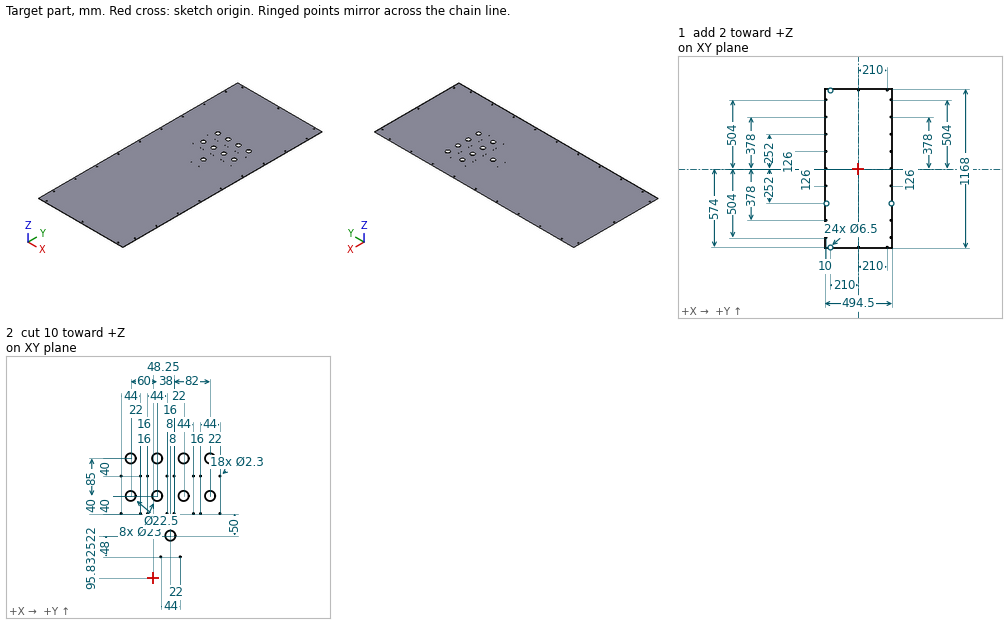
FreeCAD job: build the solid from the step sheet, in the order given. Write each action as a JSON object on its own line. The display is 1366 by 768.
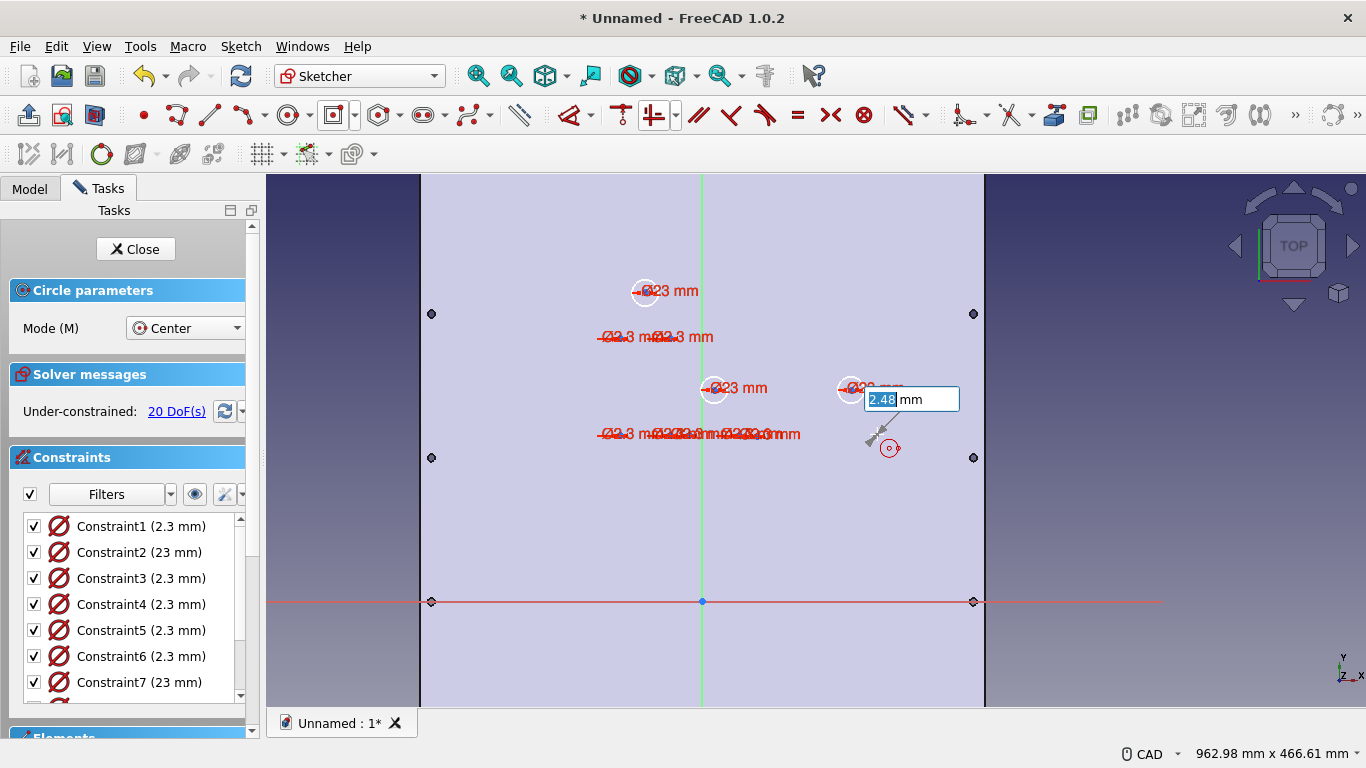
{"action": "type", "text": "2.3"}
{"action": "key", "text": "Return"}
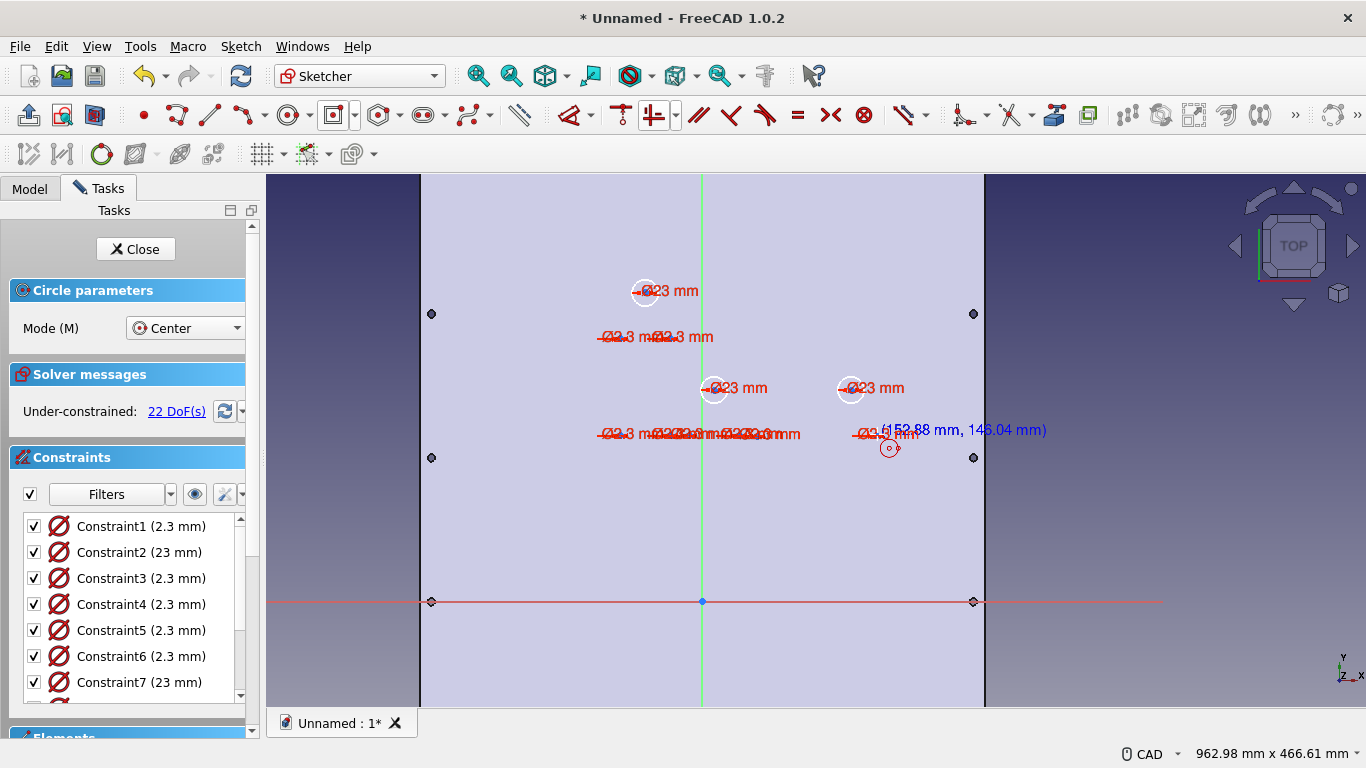
{"action": "scroll", "coordinate": [826, 435], "scroll_direction": "up", "scroll_amount": 15}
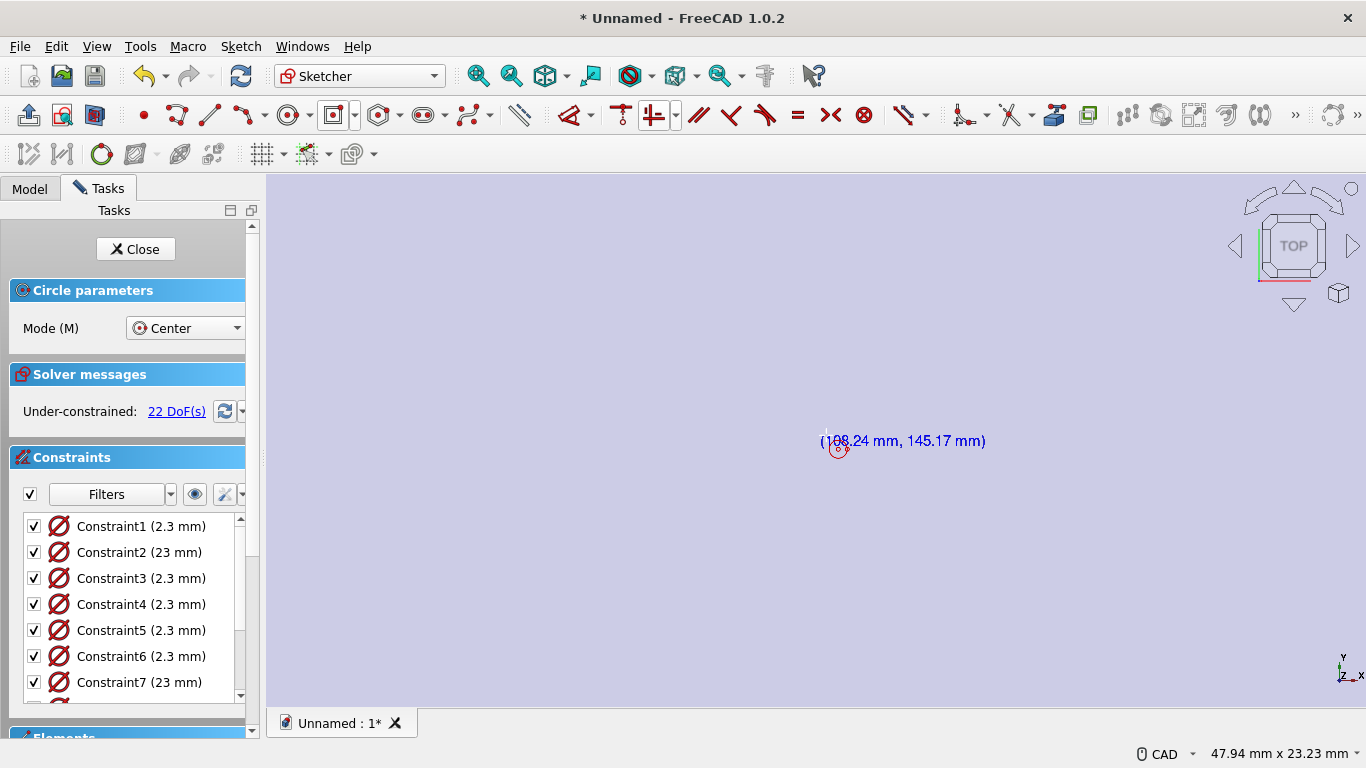
{"action": "scroll", "coordinate": [826, 435], "scroll_direction": "down", "scroll_amount": 15}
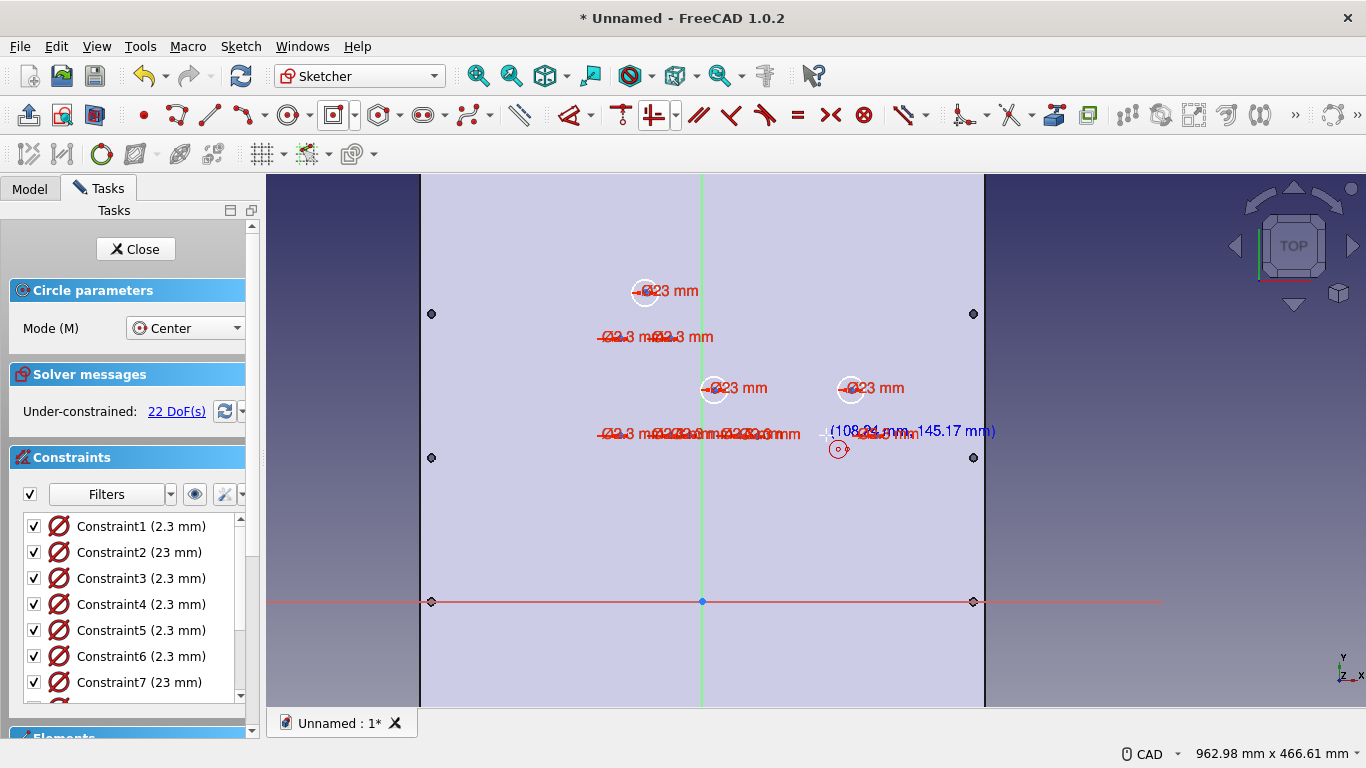
{"action": "left_click", "coordinate": [826, 435]}
{"action": "mouse_move", "coordinate": [827, 434]}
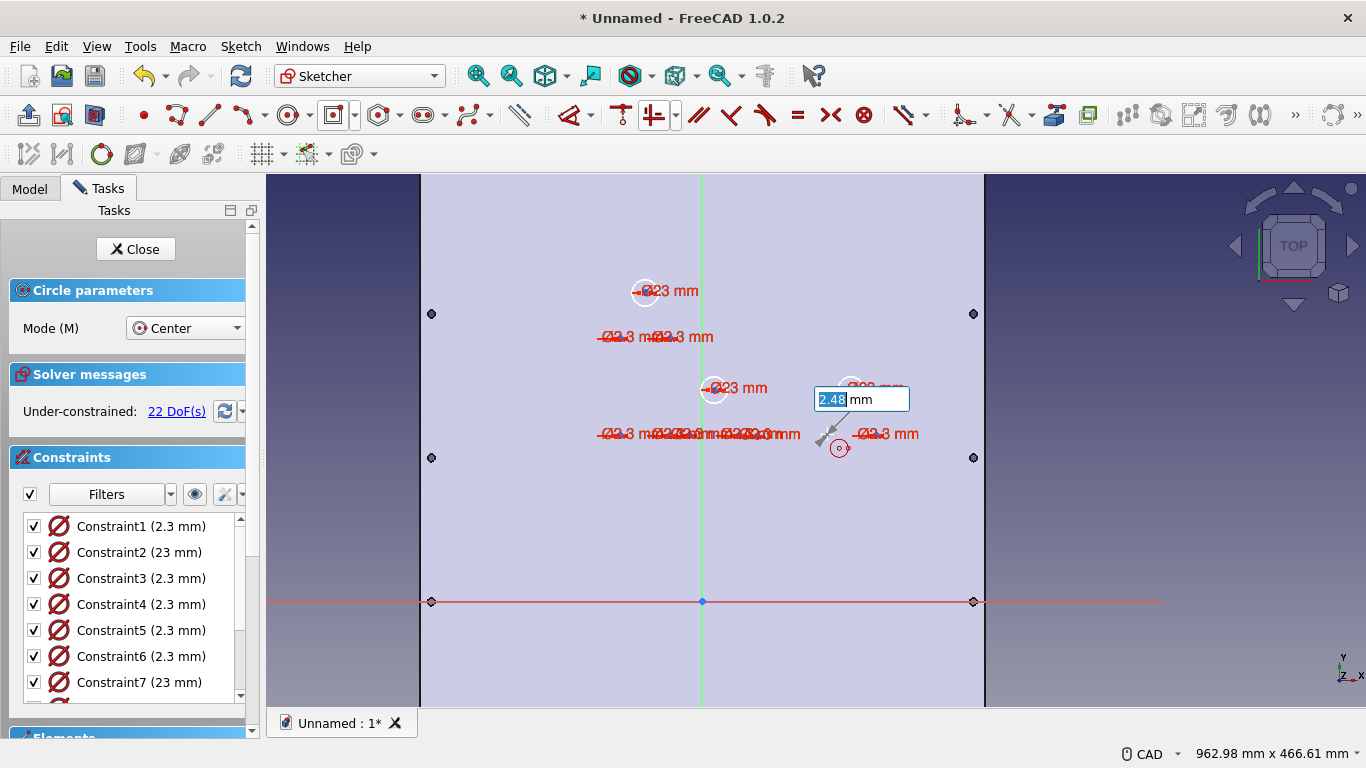
{"action": "type", "text": "2.3"}
{"action": "key", "text": "Return"}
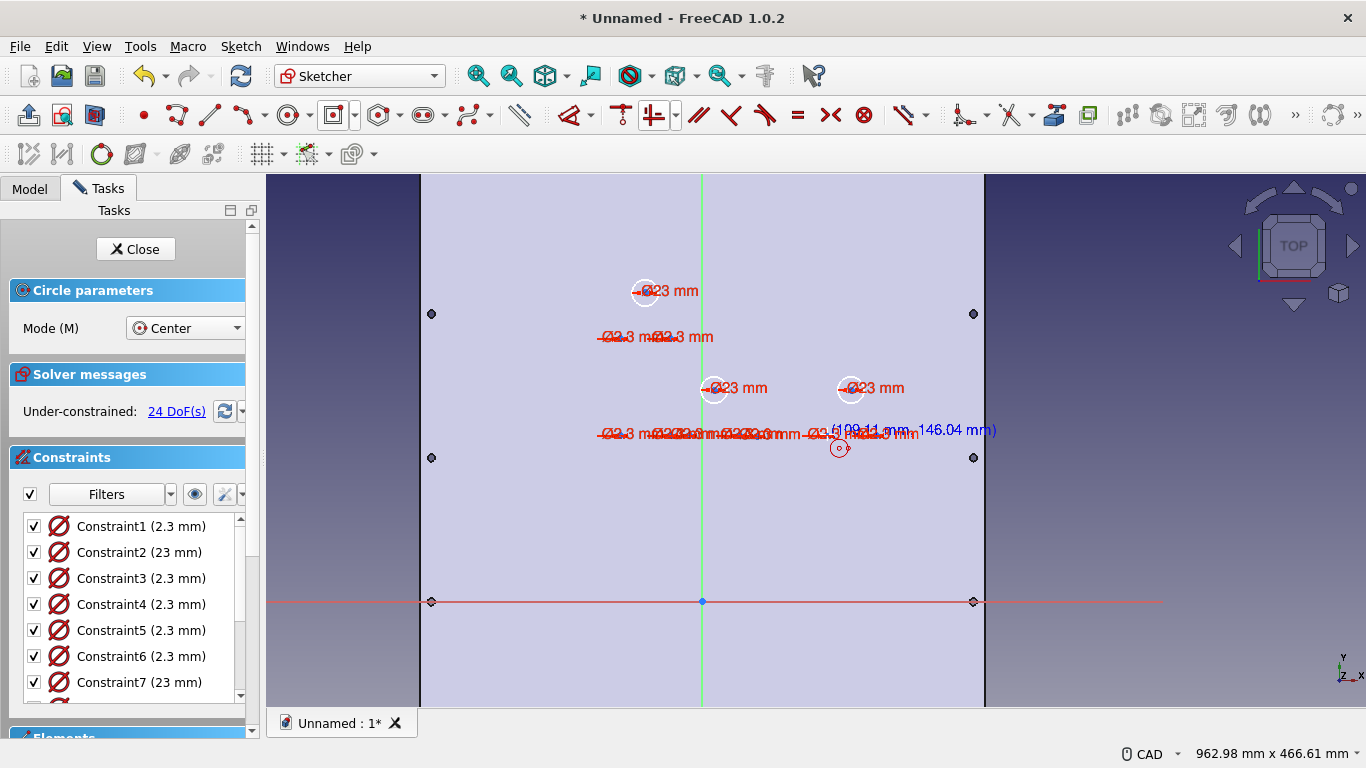
{"action": "scroll", "coordinate": [783, 390], "scroll_direction": "up", "scroll_amount": 3}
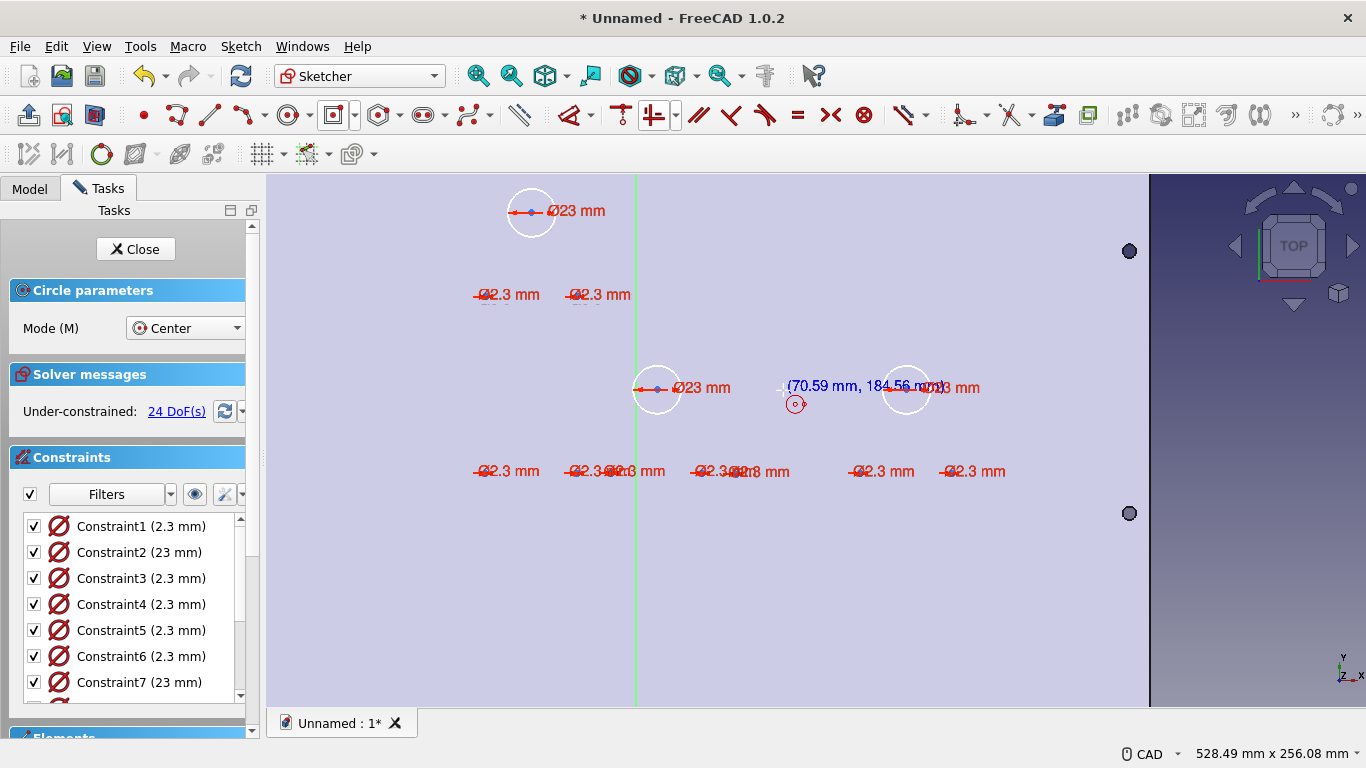
{"action": "left_click", "coordinate": [782, 389]}
{"action": "mouse_move", "coordinate": [799, 372]}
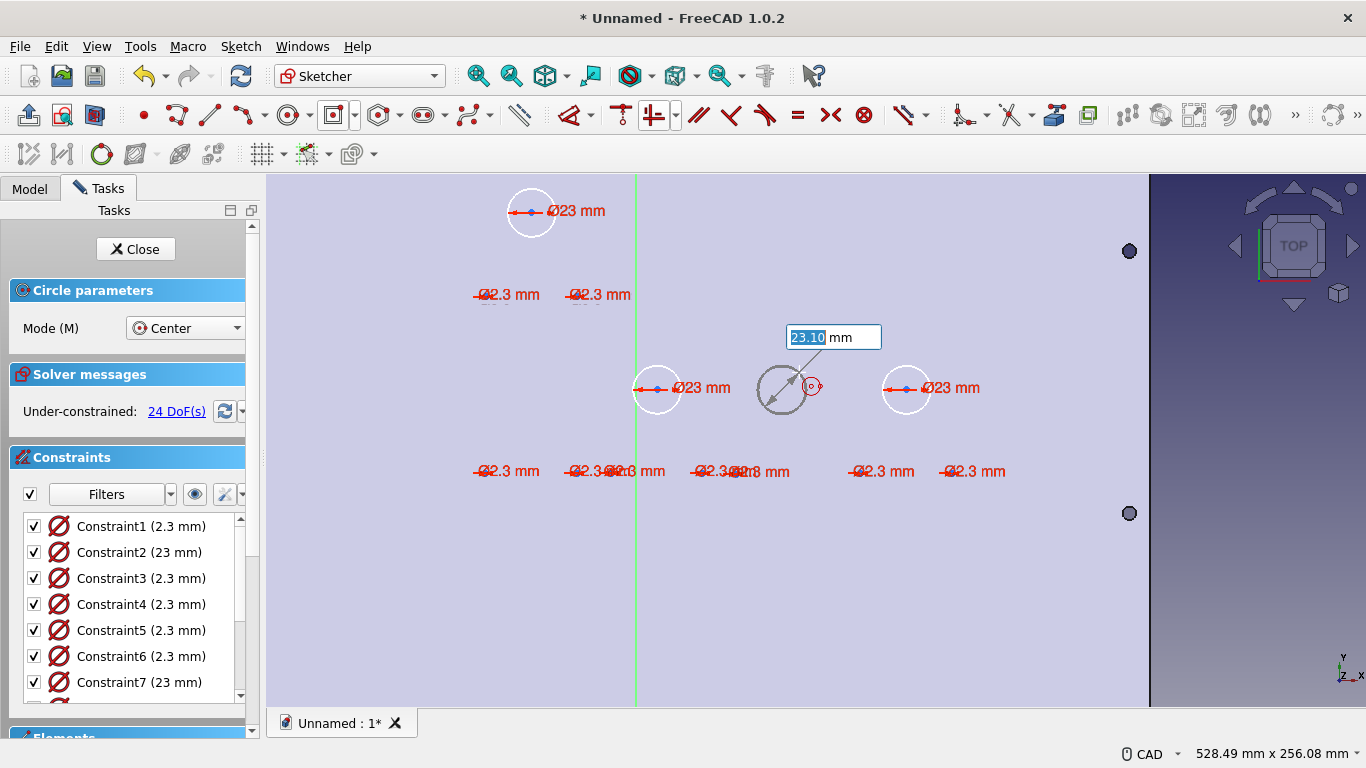
{"action": "type", "text": "23"}
{"action": "key", "text": "Return"}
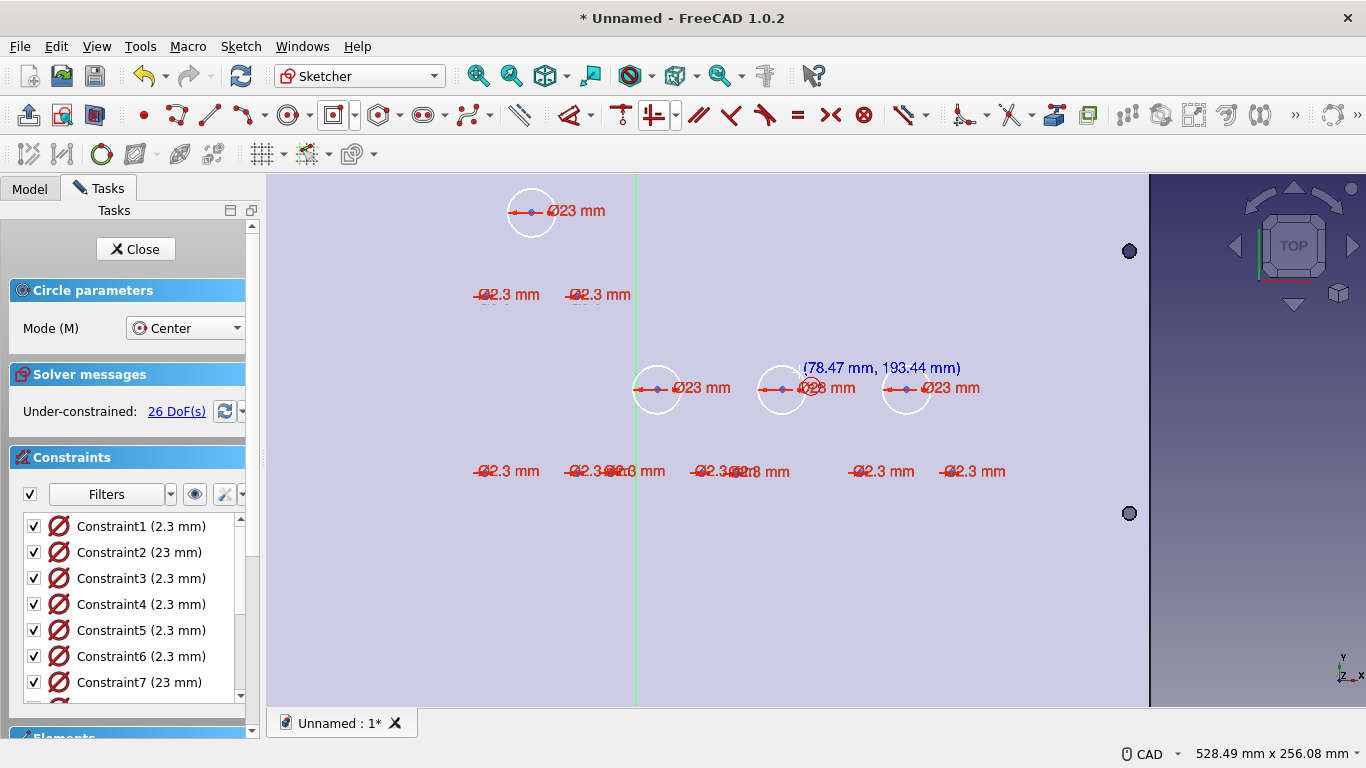
{"action": "scroll", "coordinate": [828, 472], "scroll_direction": "up", "scroll_amount": 12}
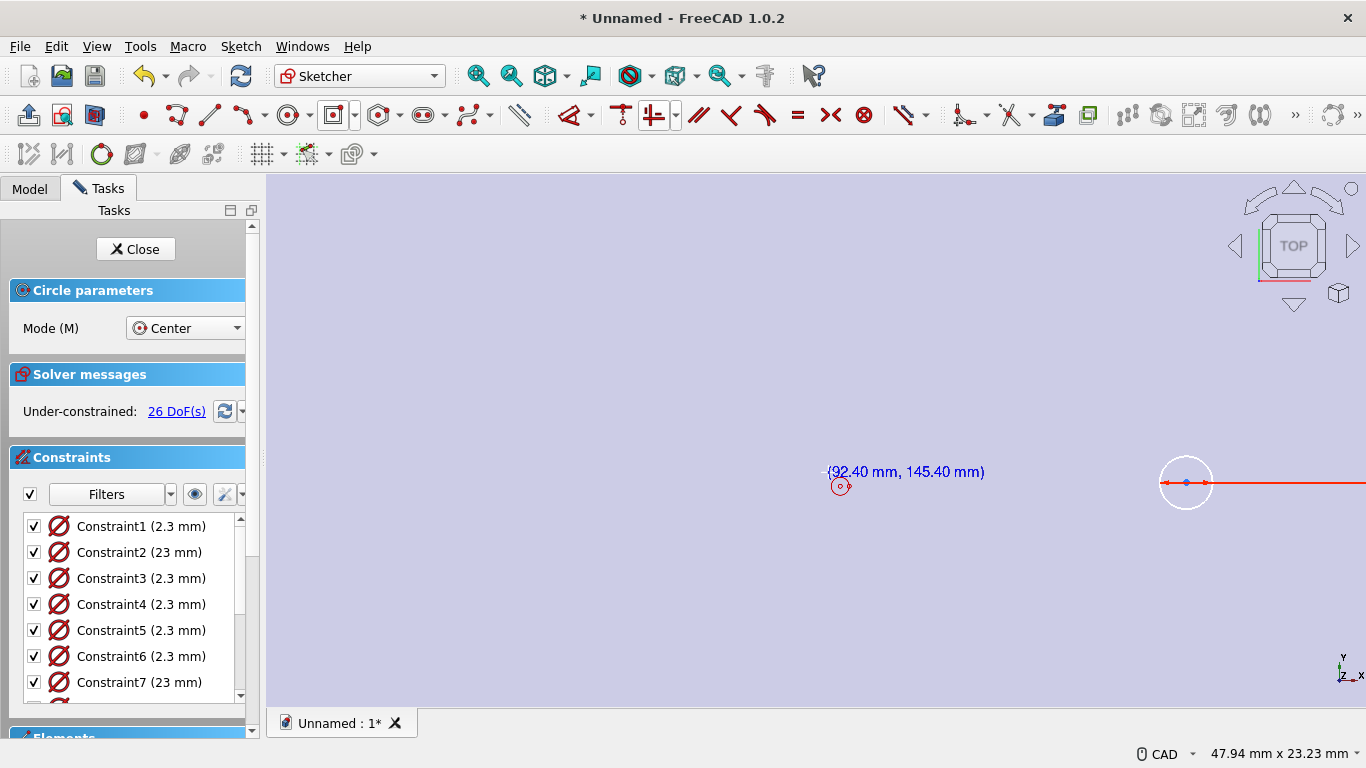
{"action": "scroll", "coordinate": [806, 433], "scroll_direction": "down", "scroll_amount": 15}